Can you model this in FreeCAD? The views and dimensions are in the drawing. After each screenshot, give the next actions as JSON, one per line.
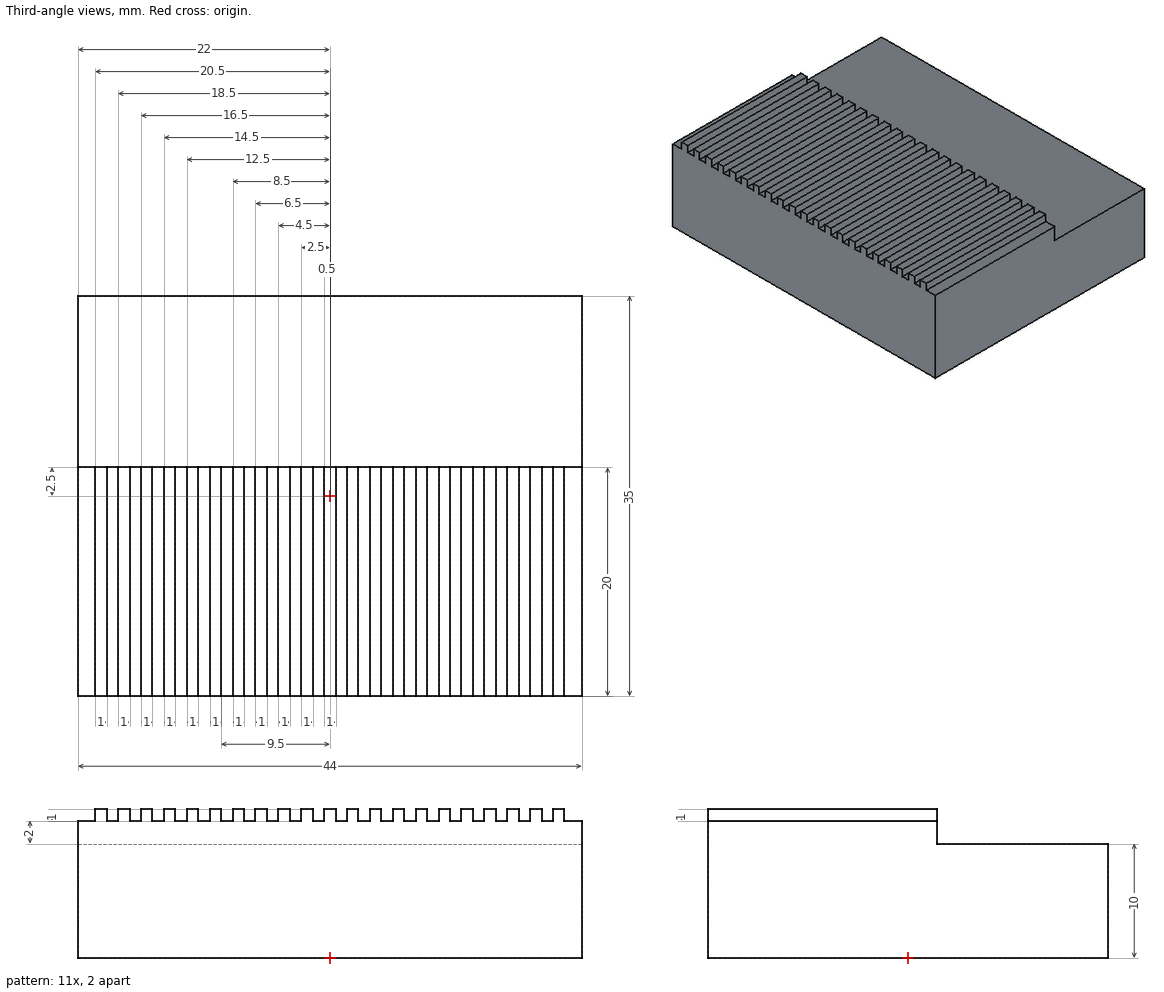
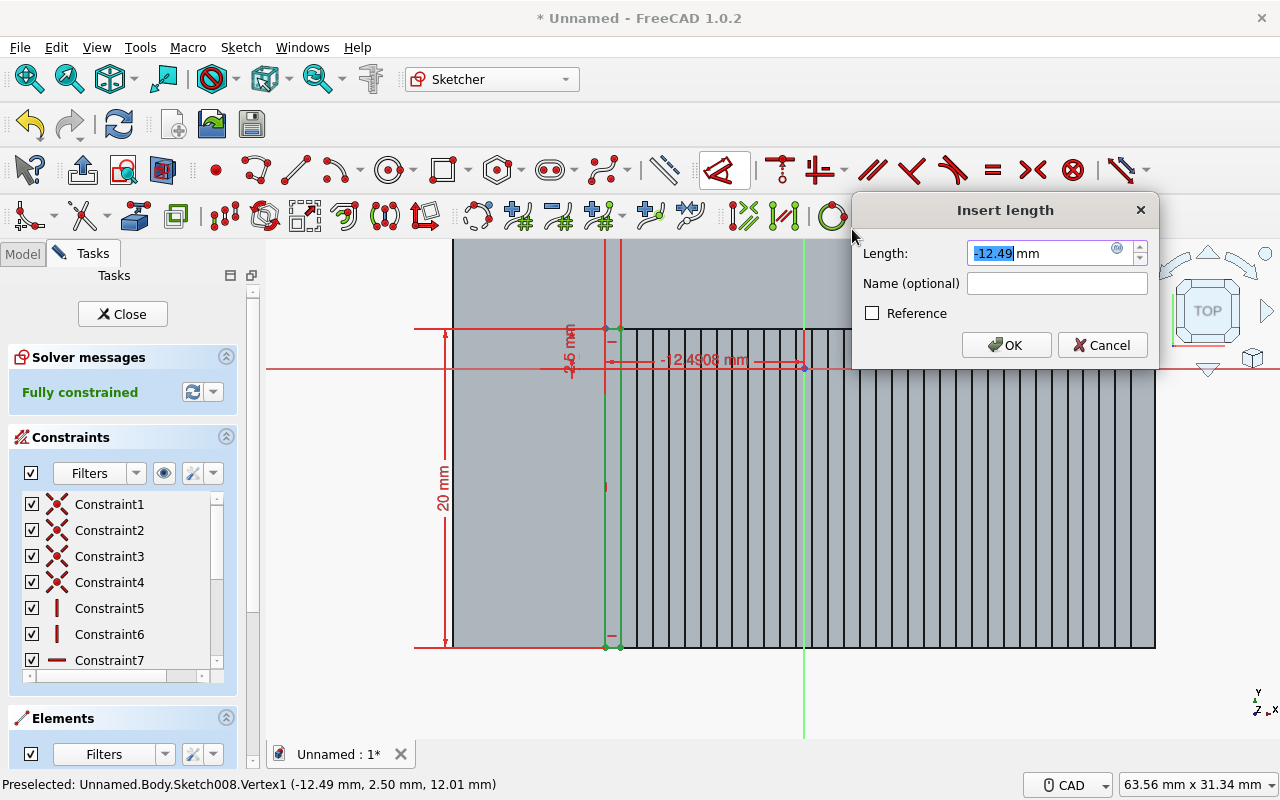
{"action": "type", "text": "-12.5"}
{"action": "key", "text": "Return"}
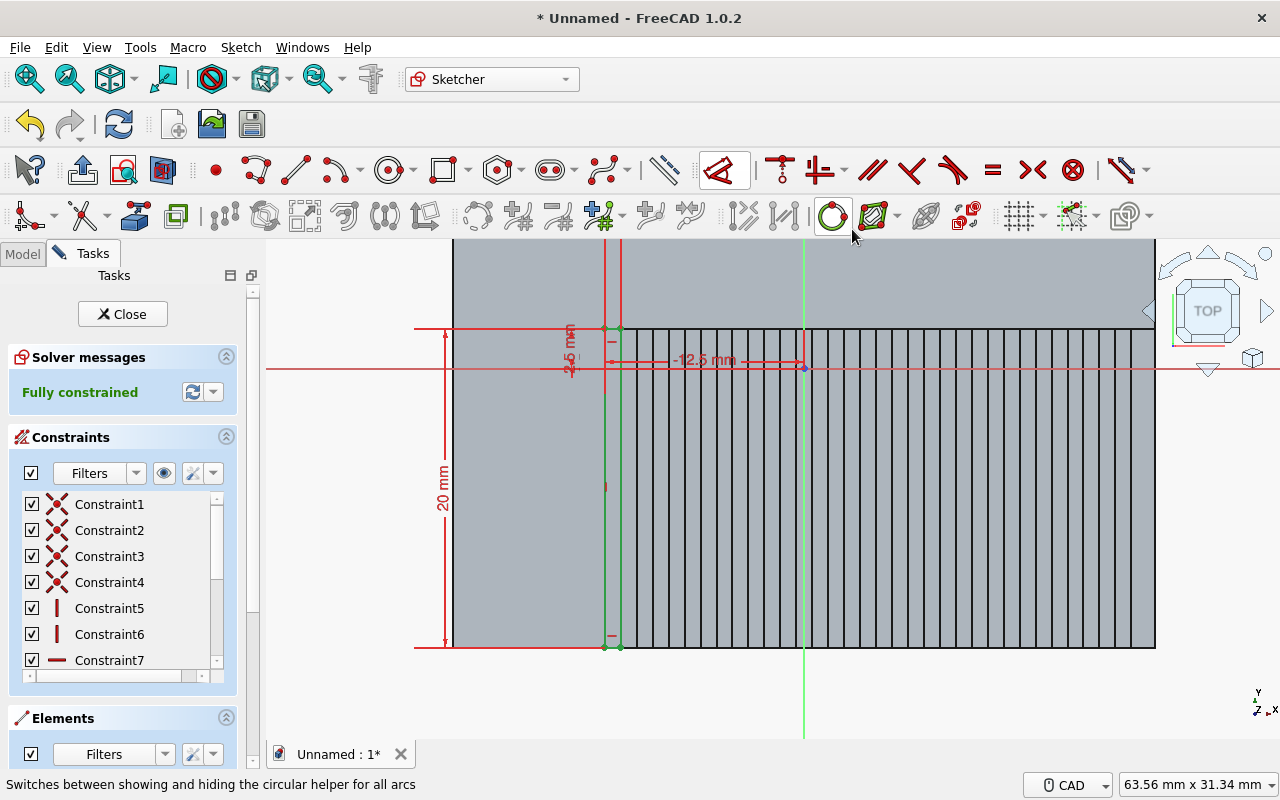
{"action": "left_click", "coordinate": [123, 314]}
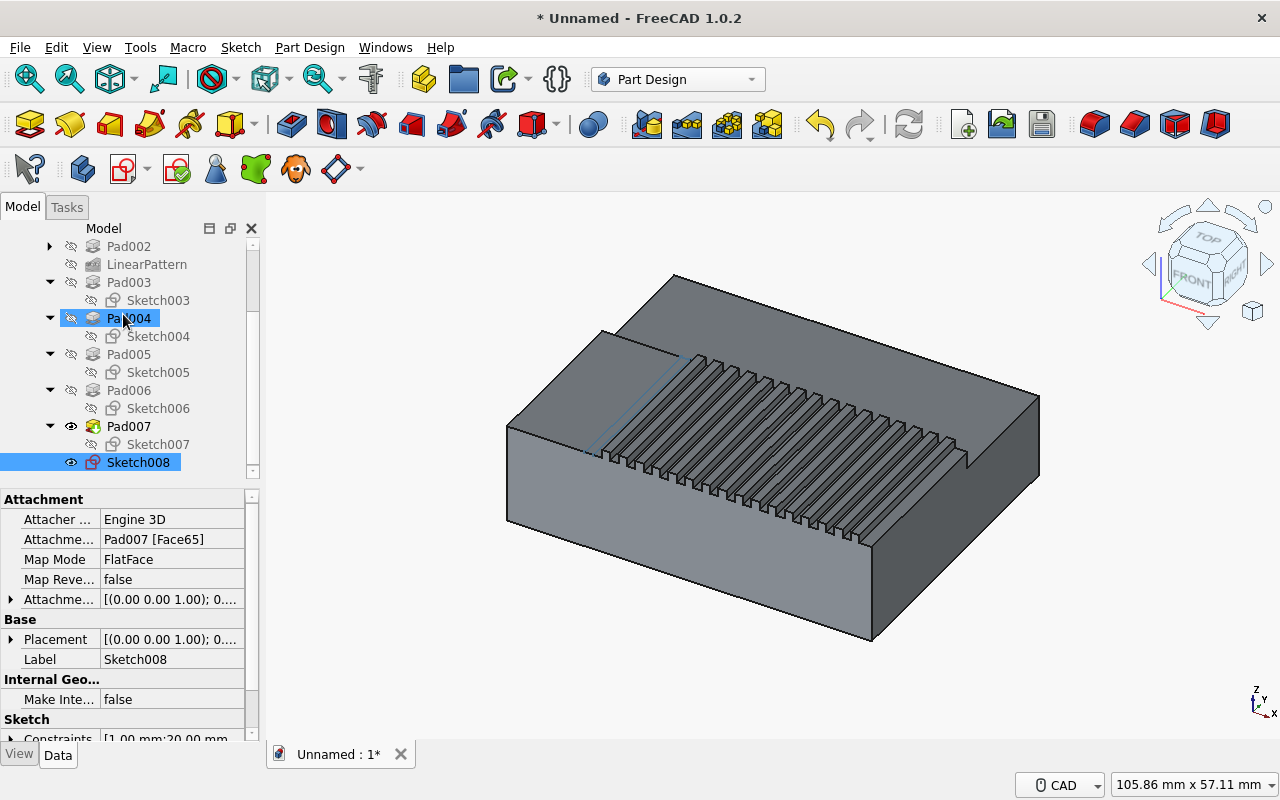
{"action": "left_click", "coordinate": [30, 124]}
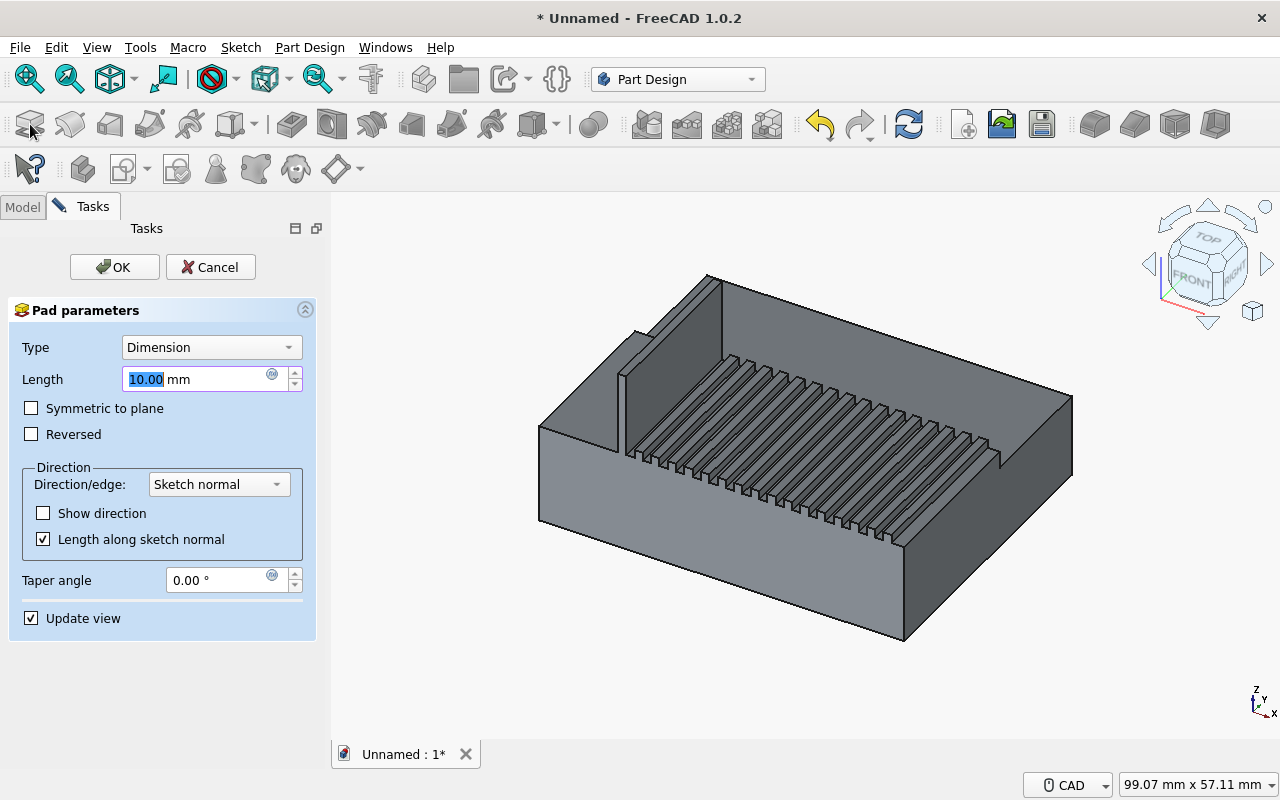
{"action": "type", "text": "1"}
{"action": "key", "text": "Tab"}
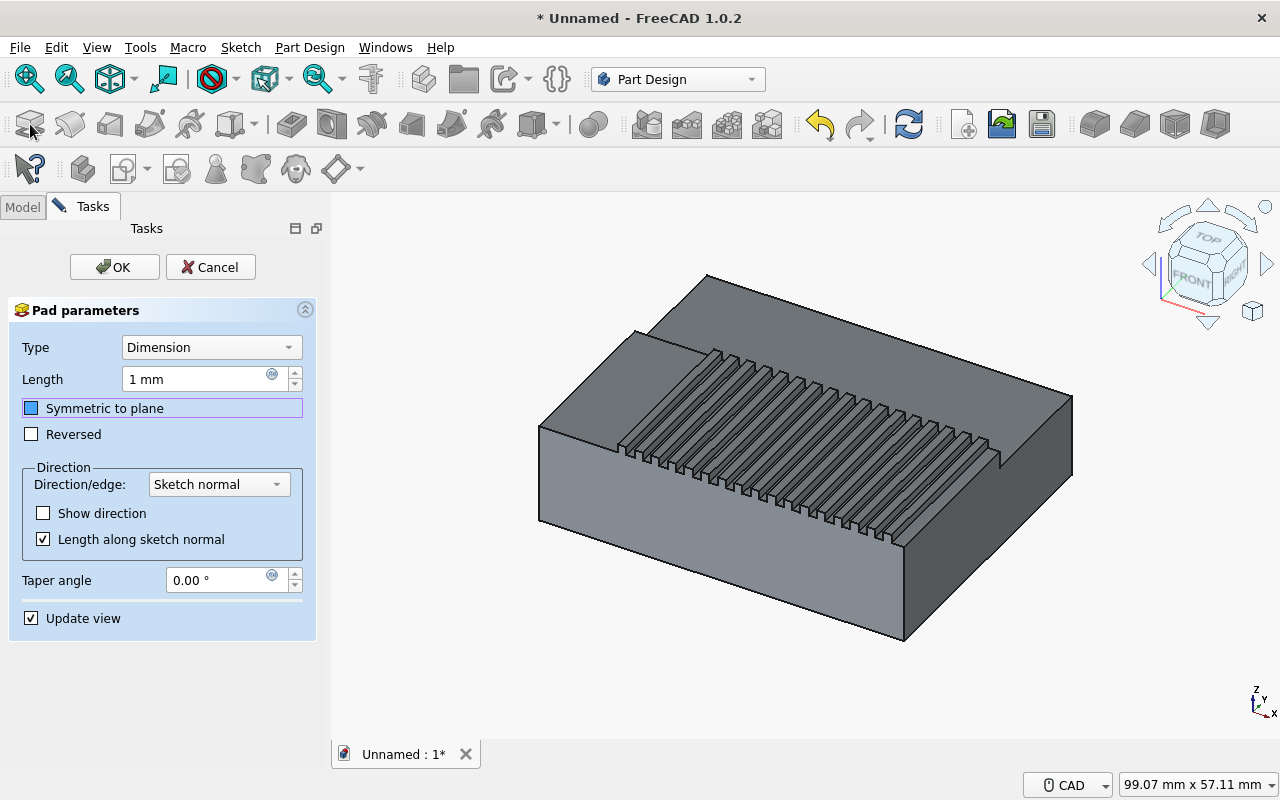
{"action": "left_click", "coordinate": [115, 267]}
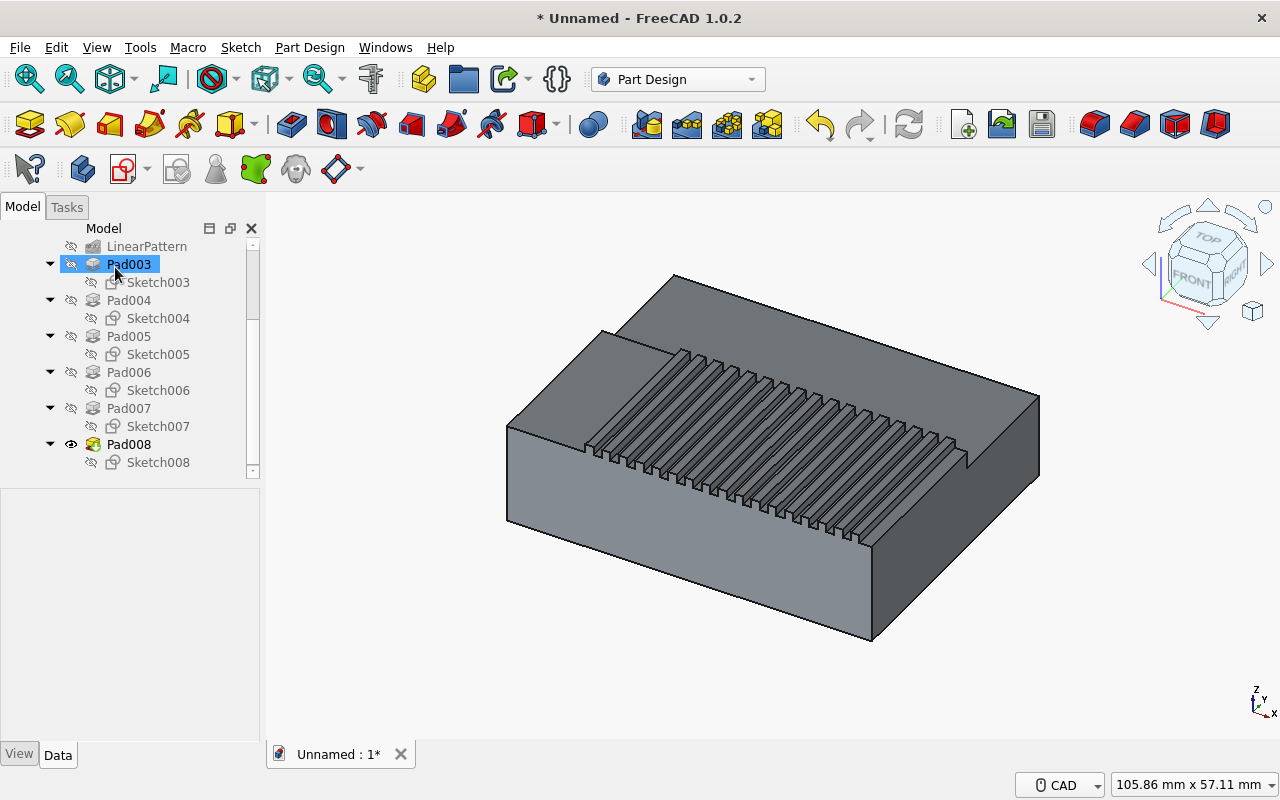
{"action": "left_click", "coordinate": [608, 377]}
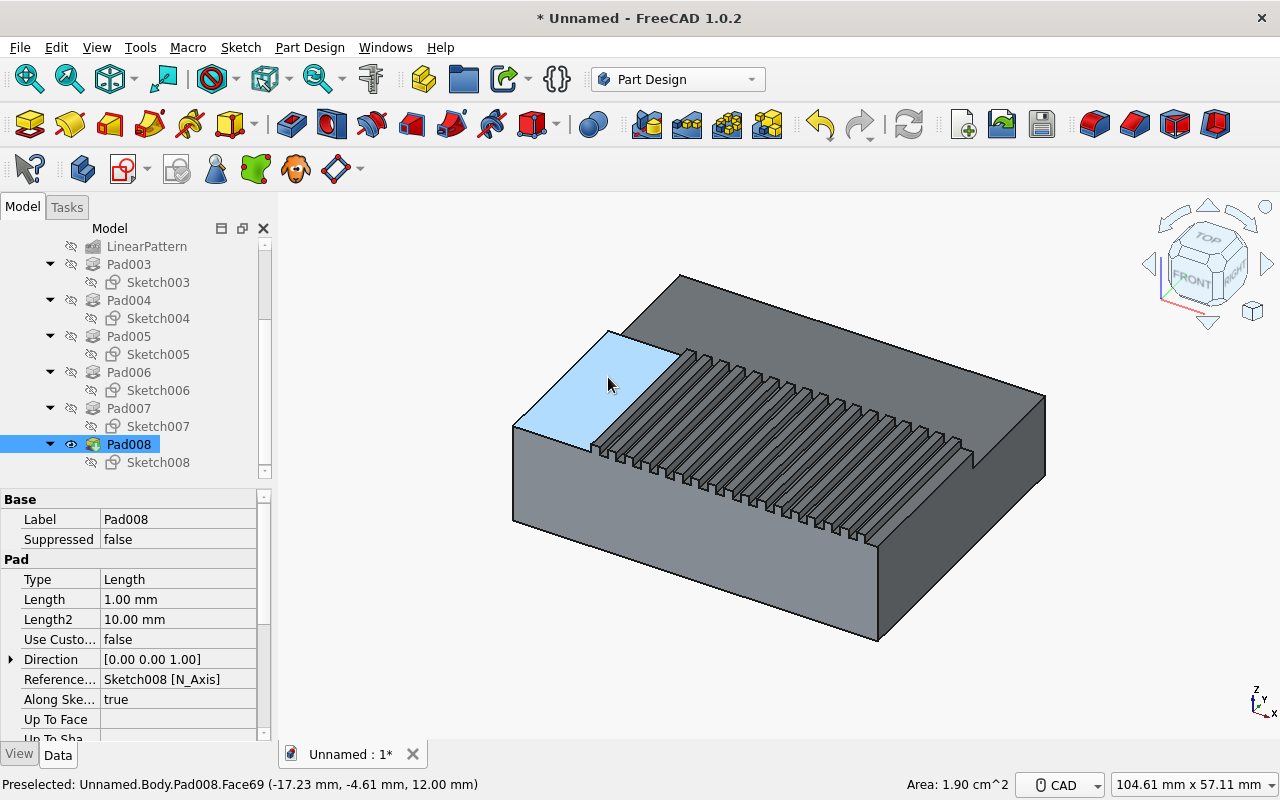
{"action": "left_click", "coordinate": [124, 170]}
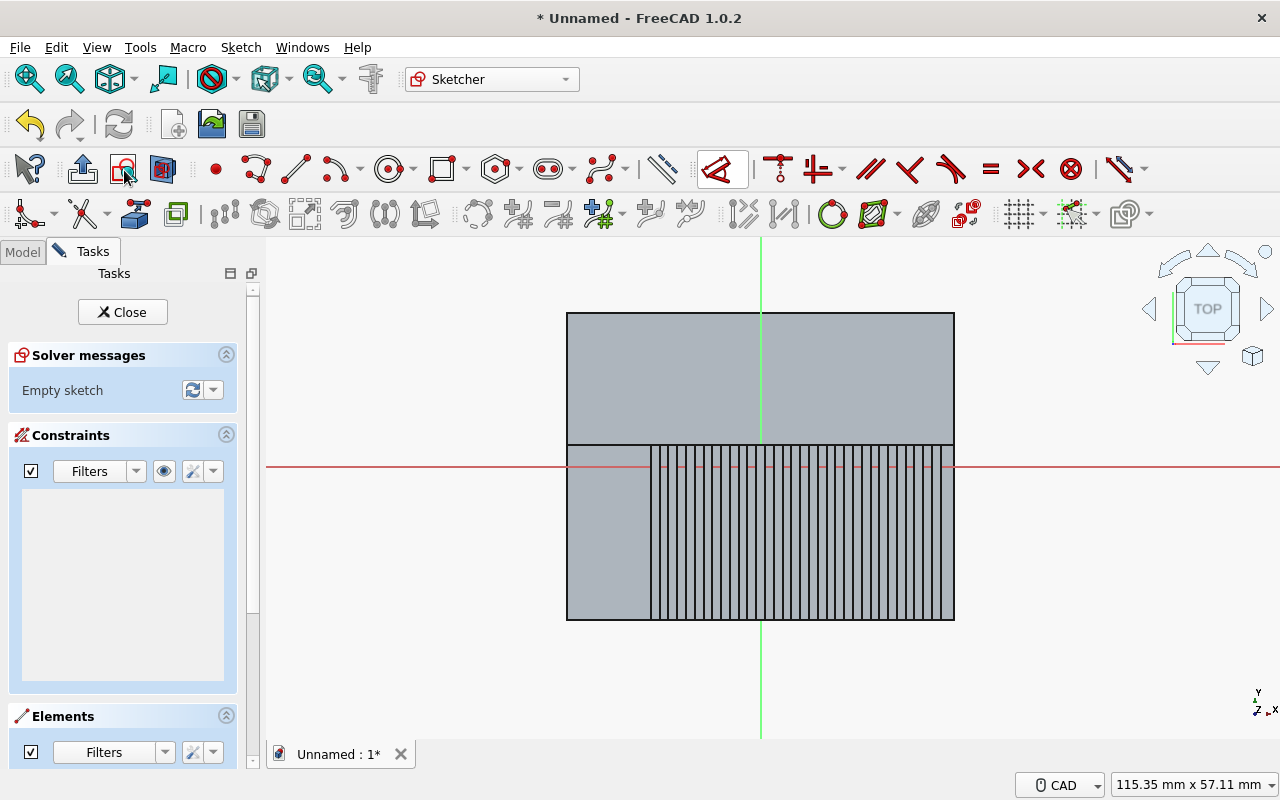
{"action": "left_click", "coordinate": [164, 170]}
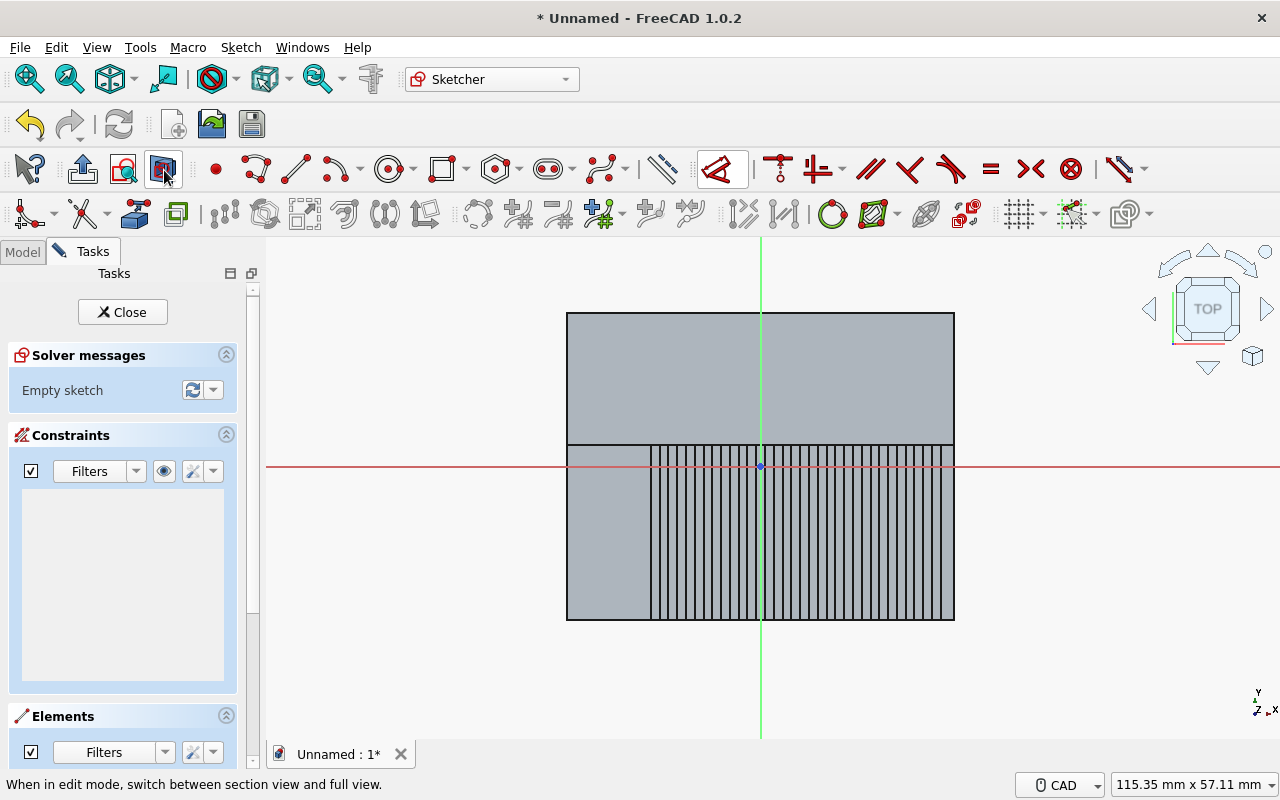
{"action": "scroll", "coordinate": [688, 587], "scroll_direction": "up", "scroll_amount": 3}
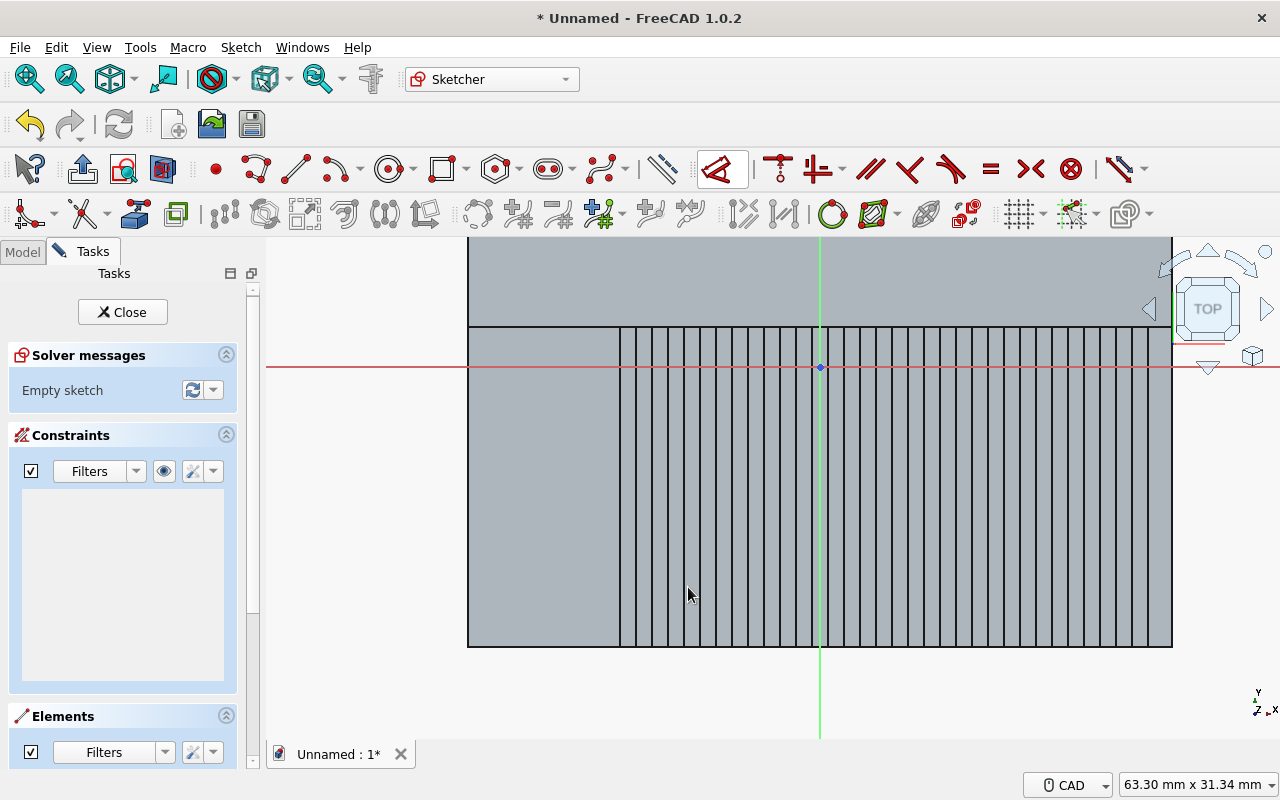
{"action": "left_click", "coordinate": [442, 170]}